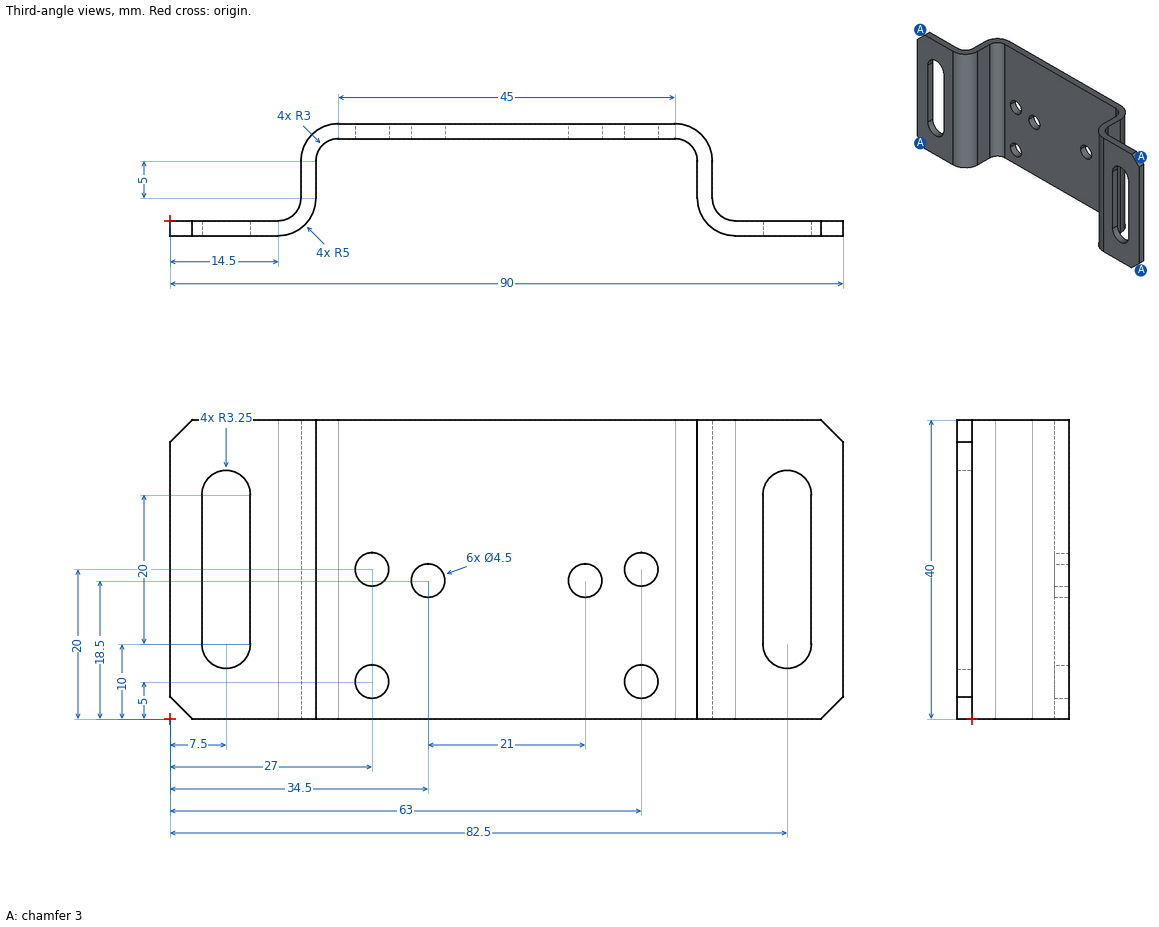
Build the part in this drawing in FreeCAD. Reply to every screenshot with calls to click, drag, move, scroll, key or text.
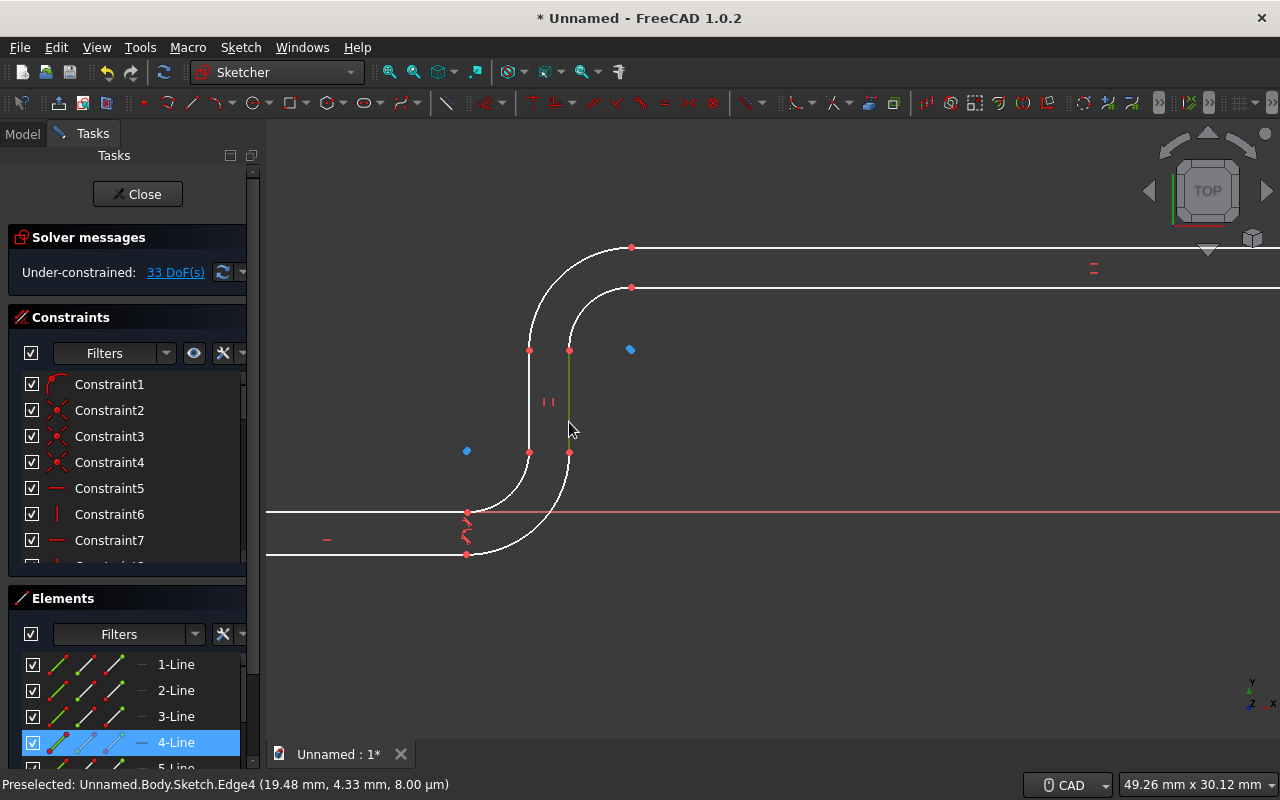
click(513, 544)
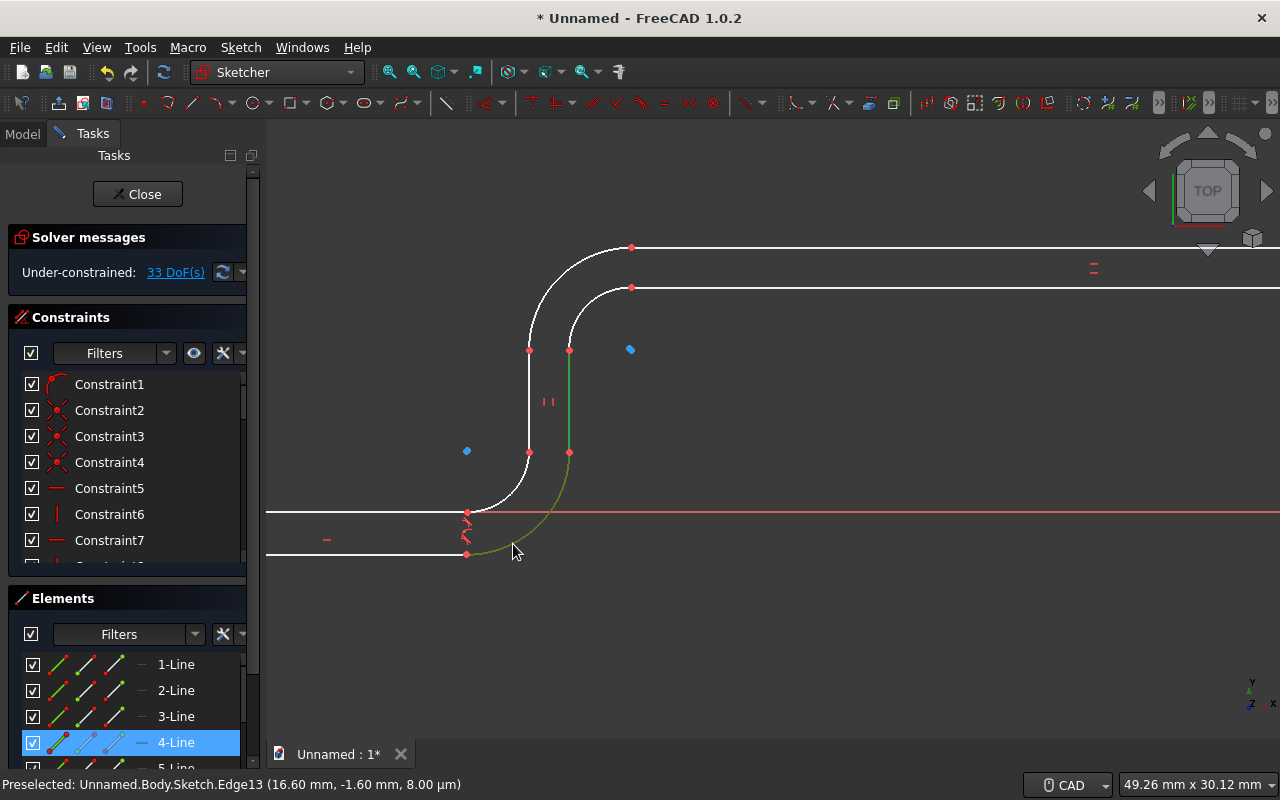
key(t)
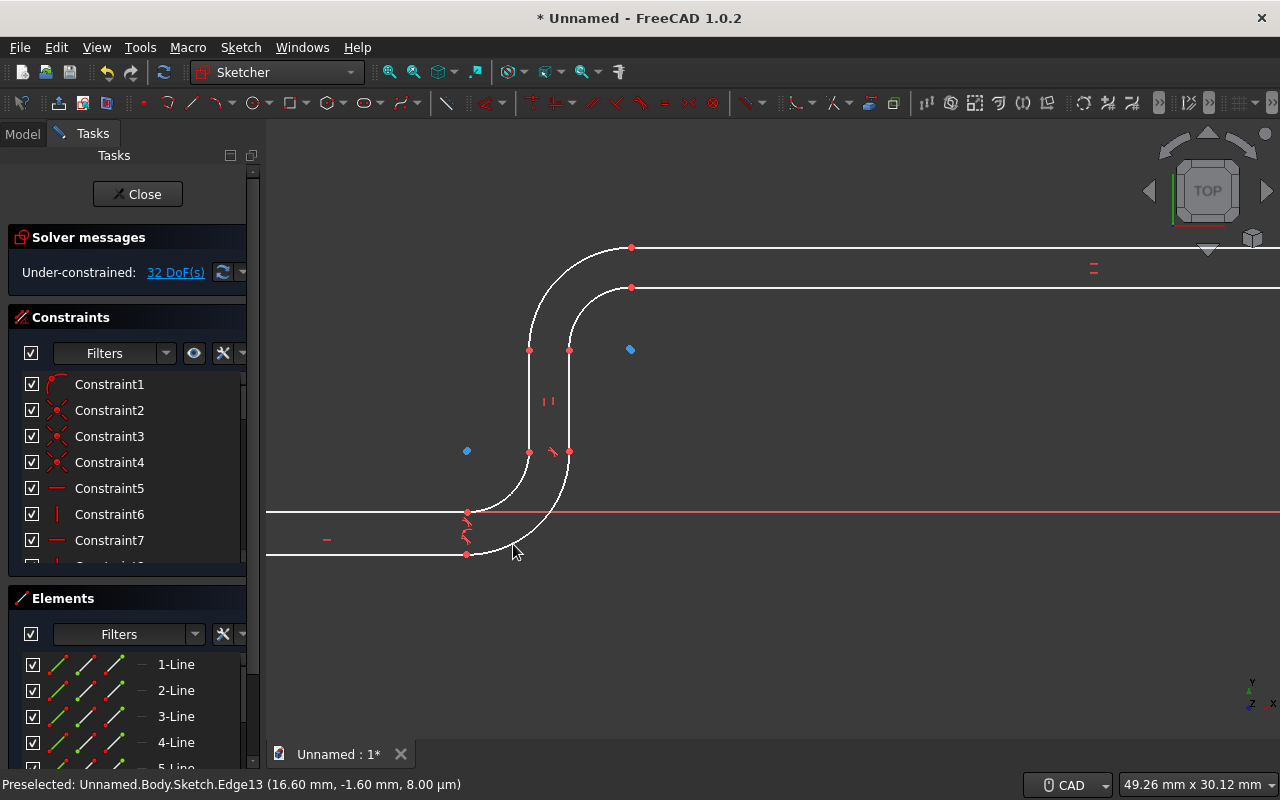
click(569, 421)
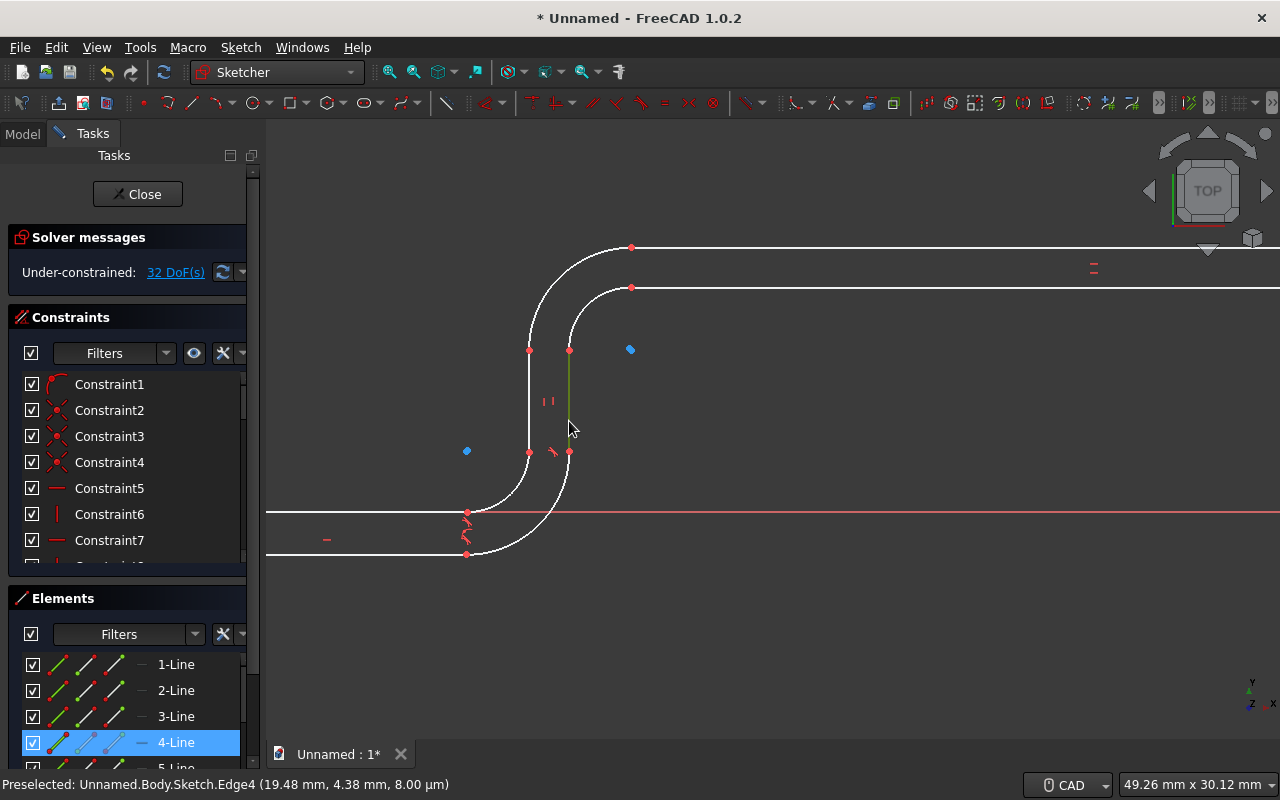
click(603, 294)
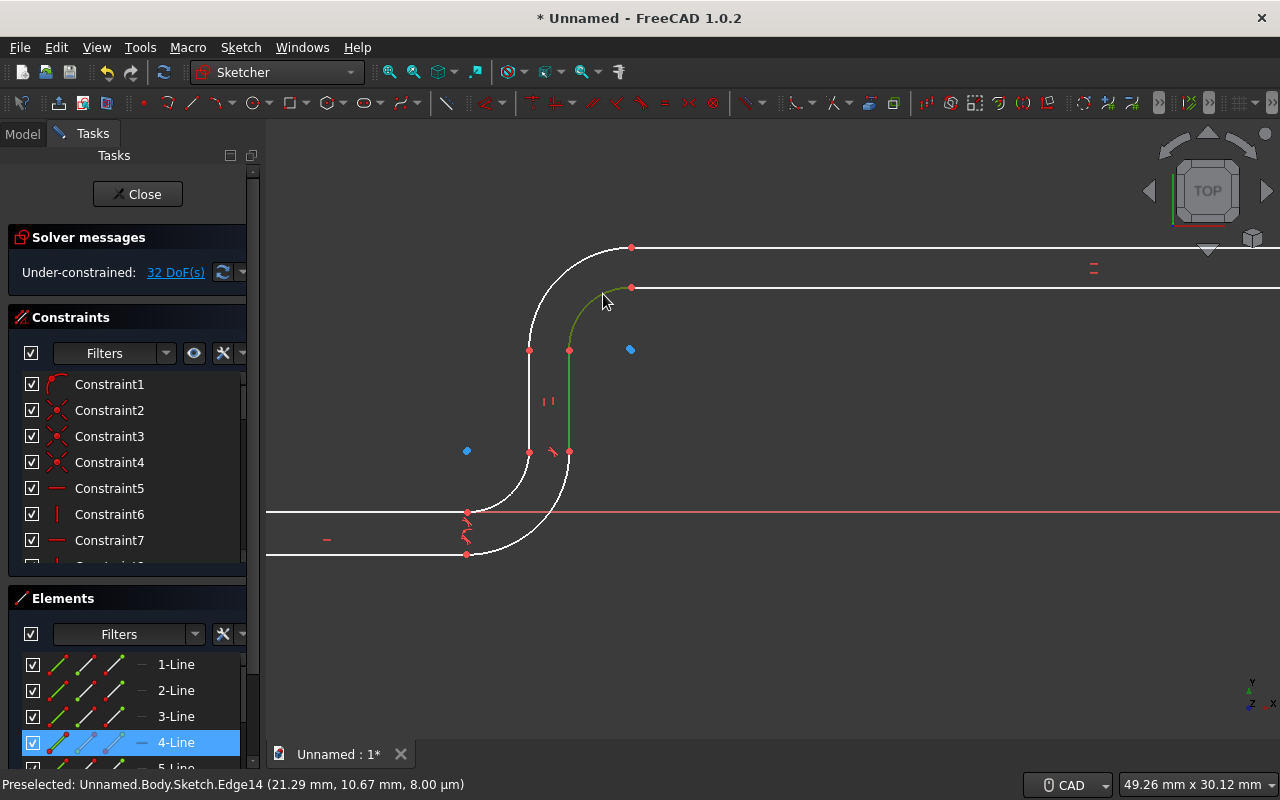
click(642, 104)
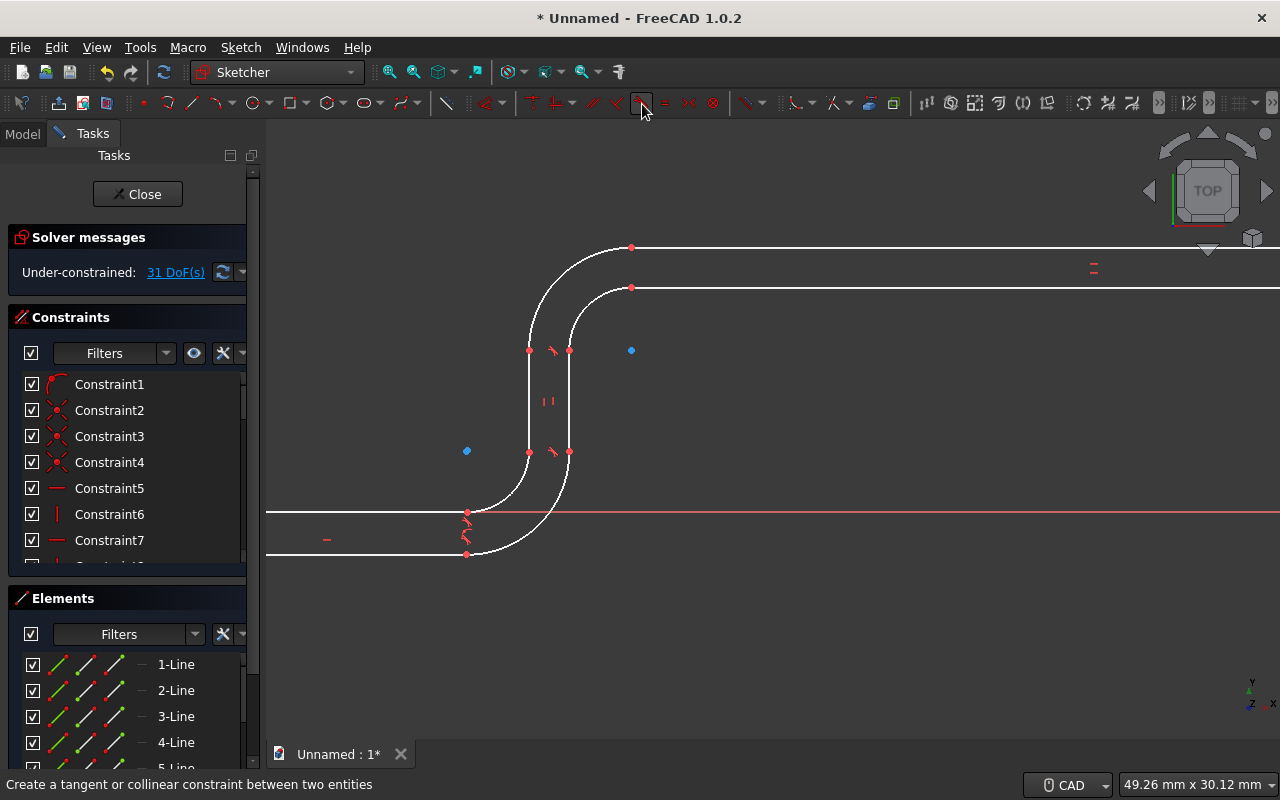
click(909, 288)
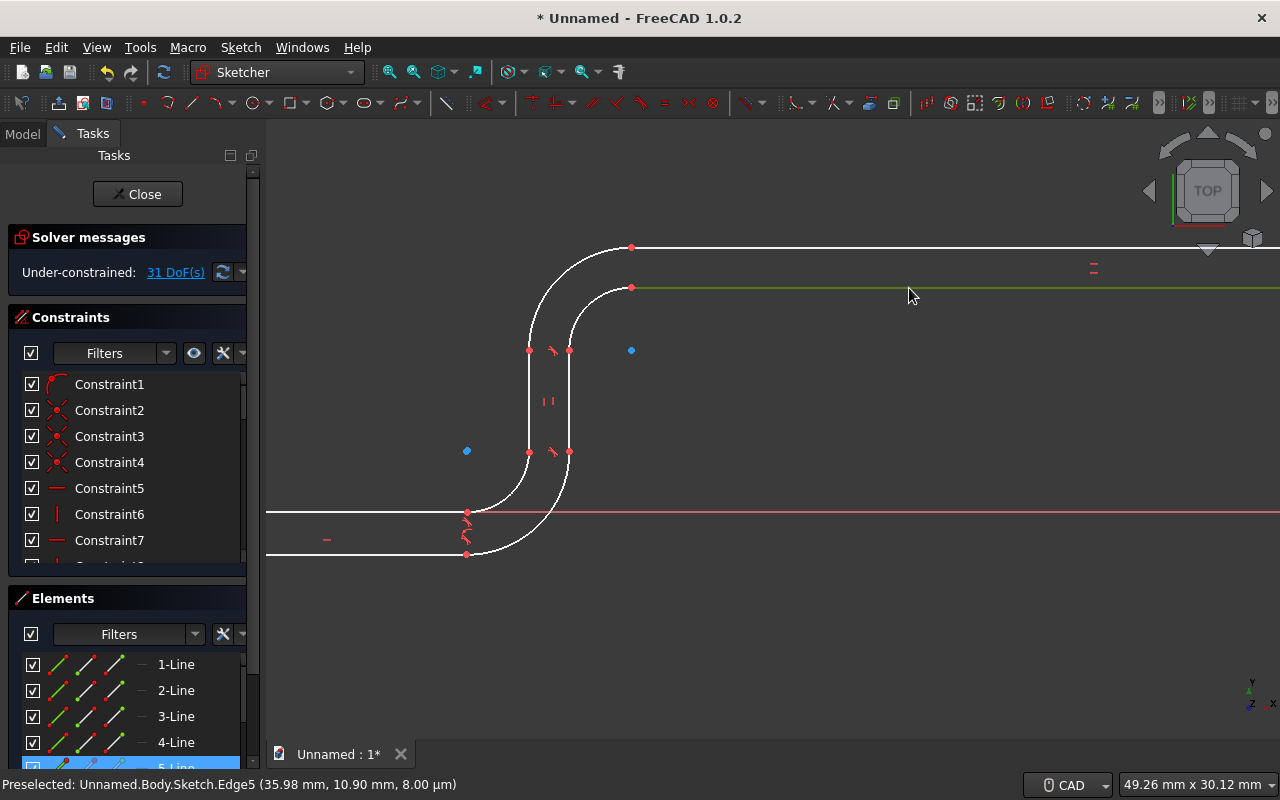
click(603, 295)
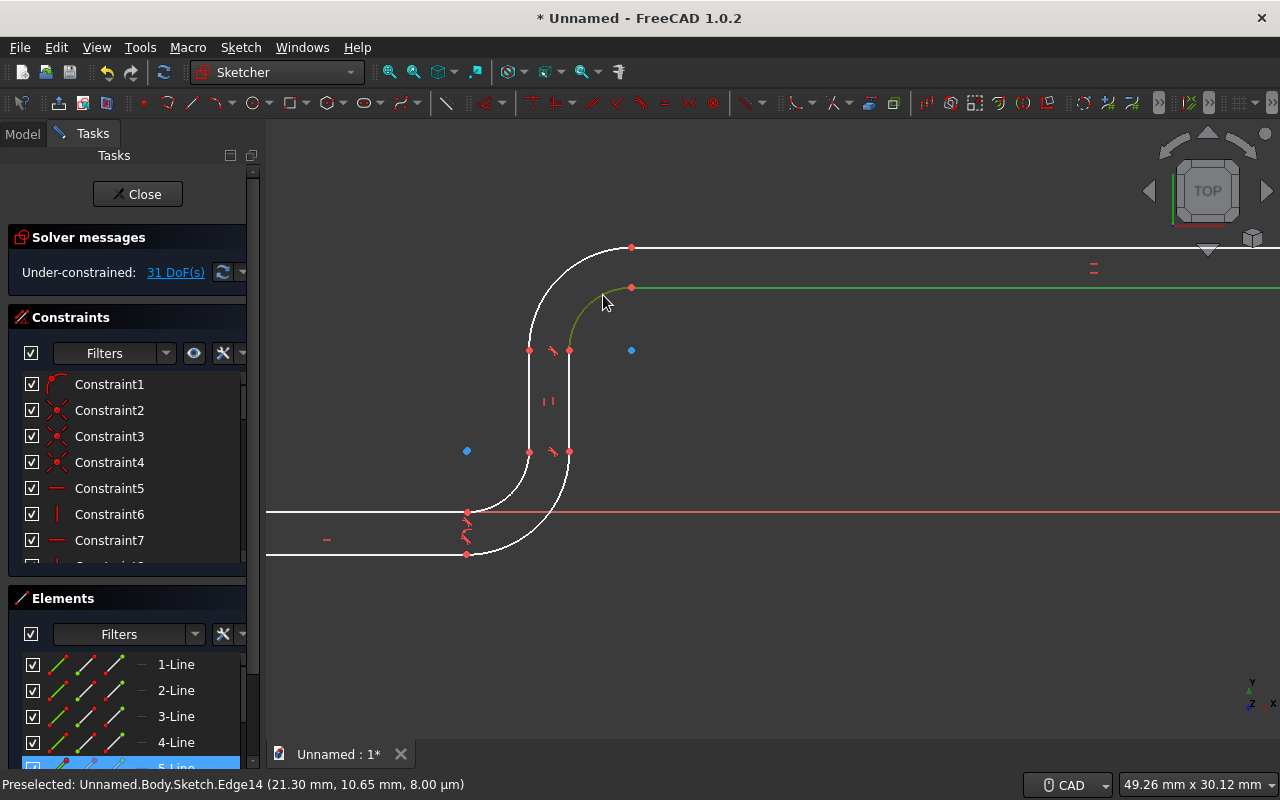
click(642, 104)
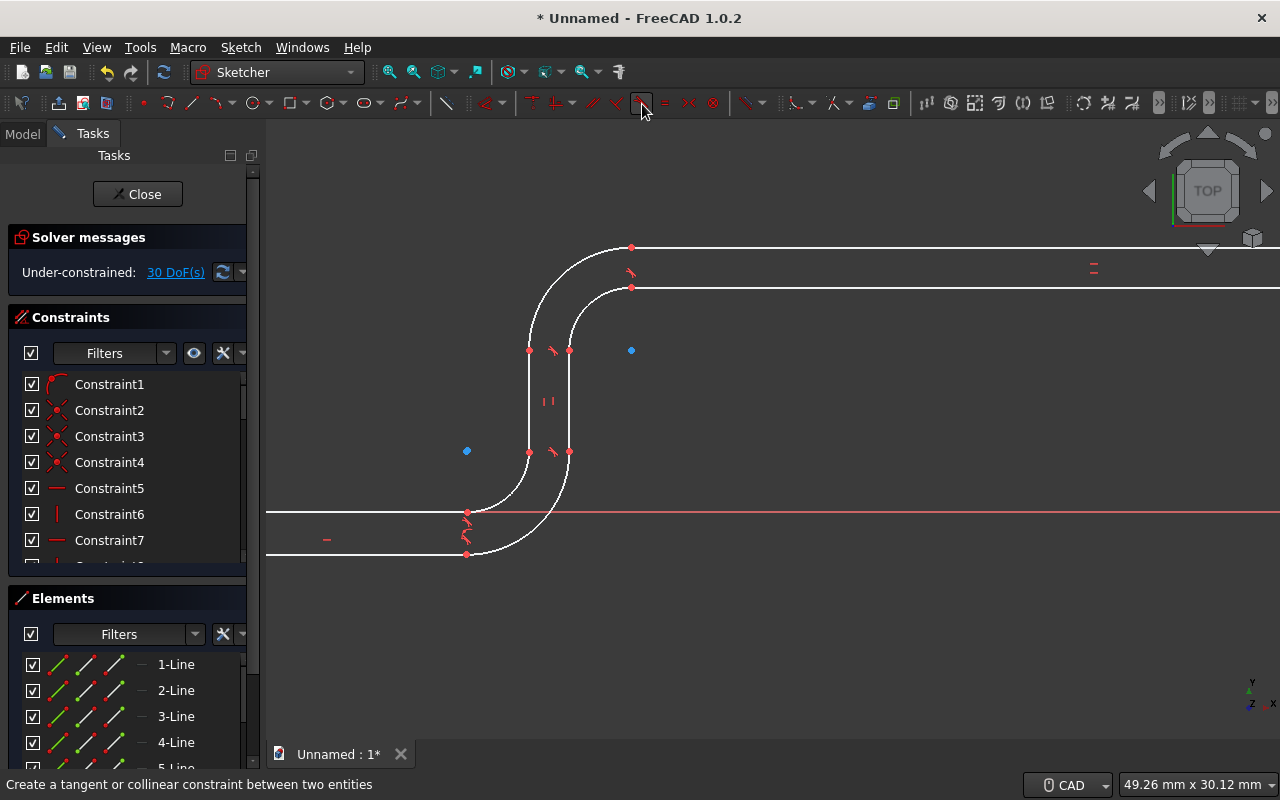
click(909, 288)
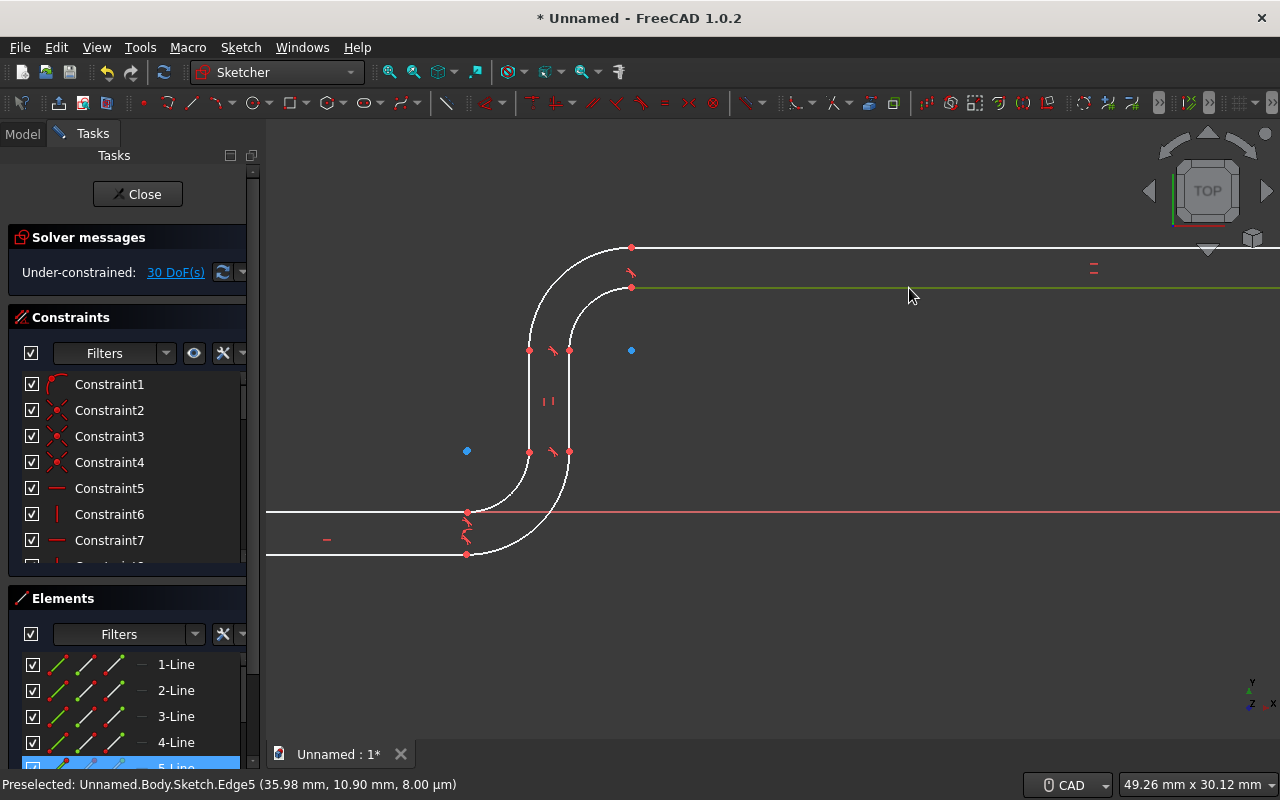
scroll(536, 442, down, 6)